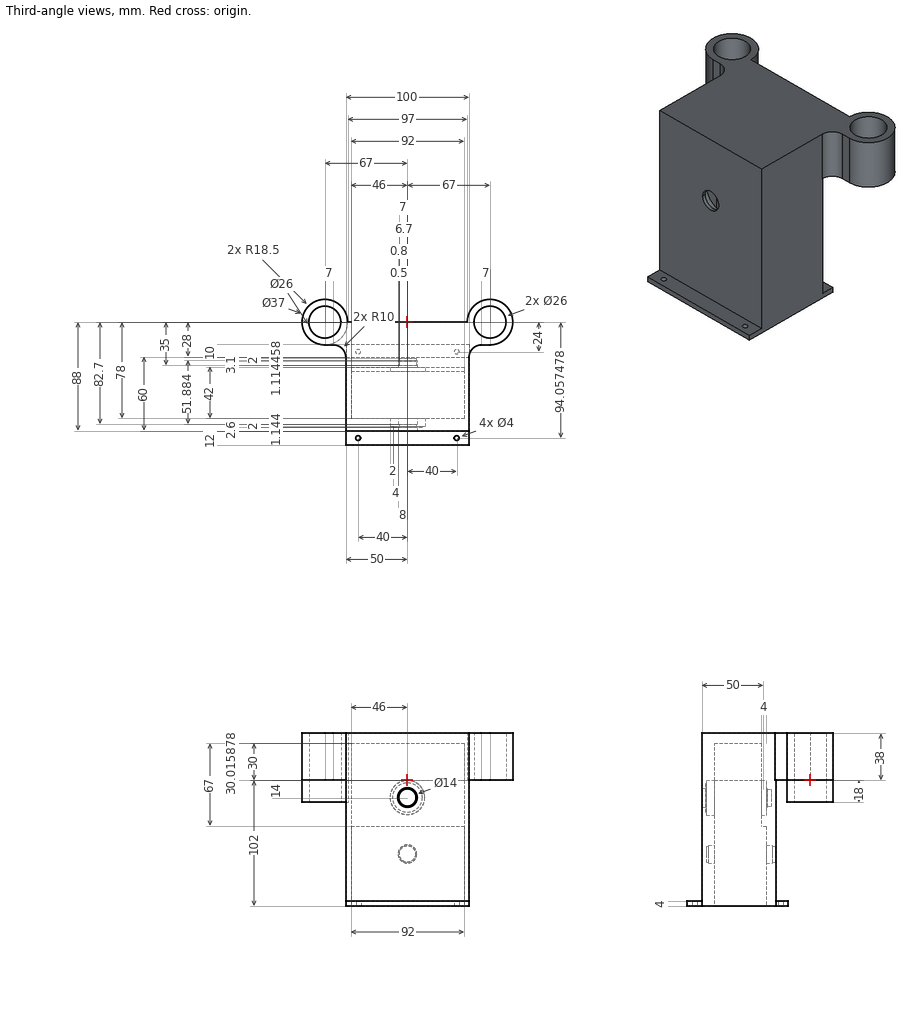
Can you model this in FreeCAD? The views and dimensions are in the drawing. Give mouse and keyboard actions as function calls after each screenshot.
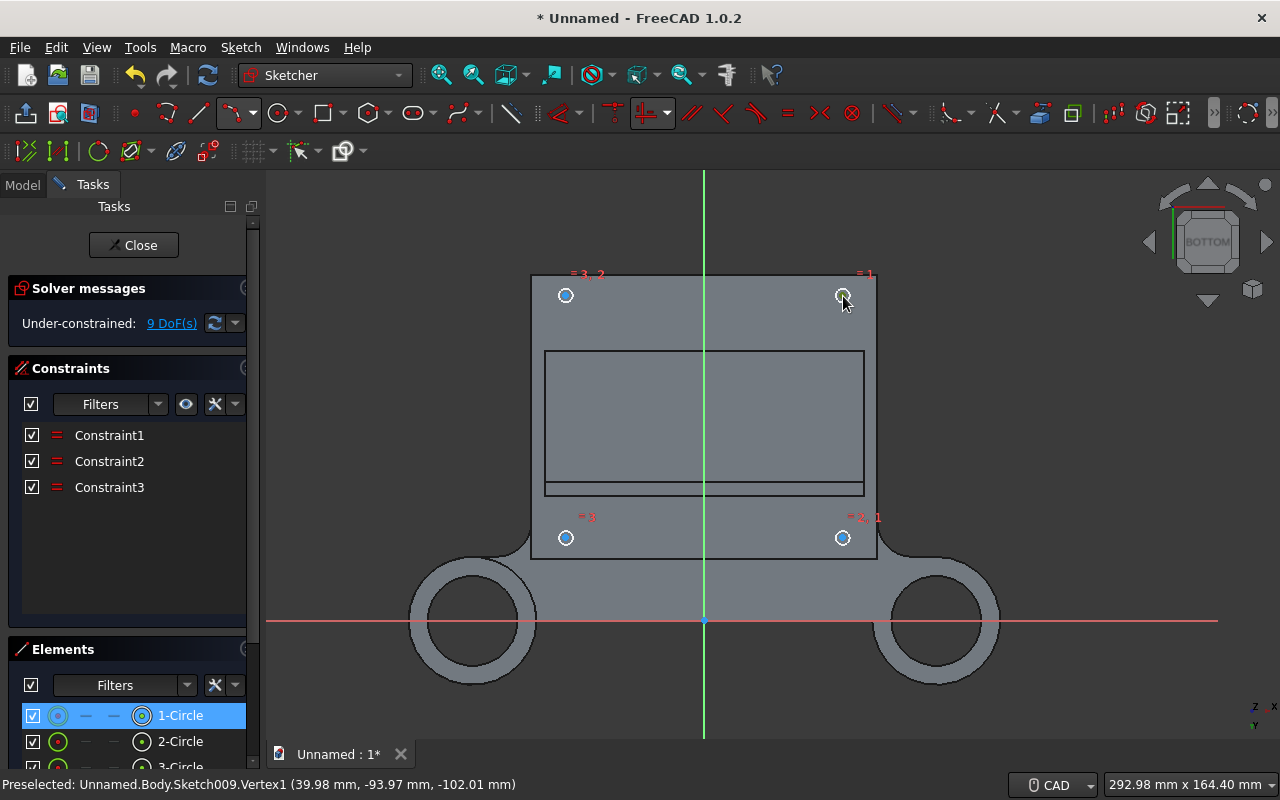
click(843, 538)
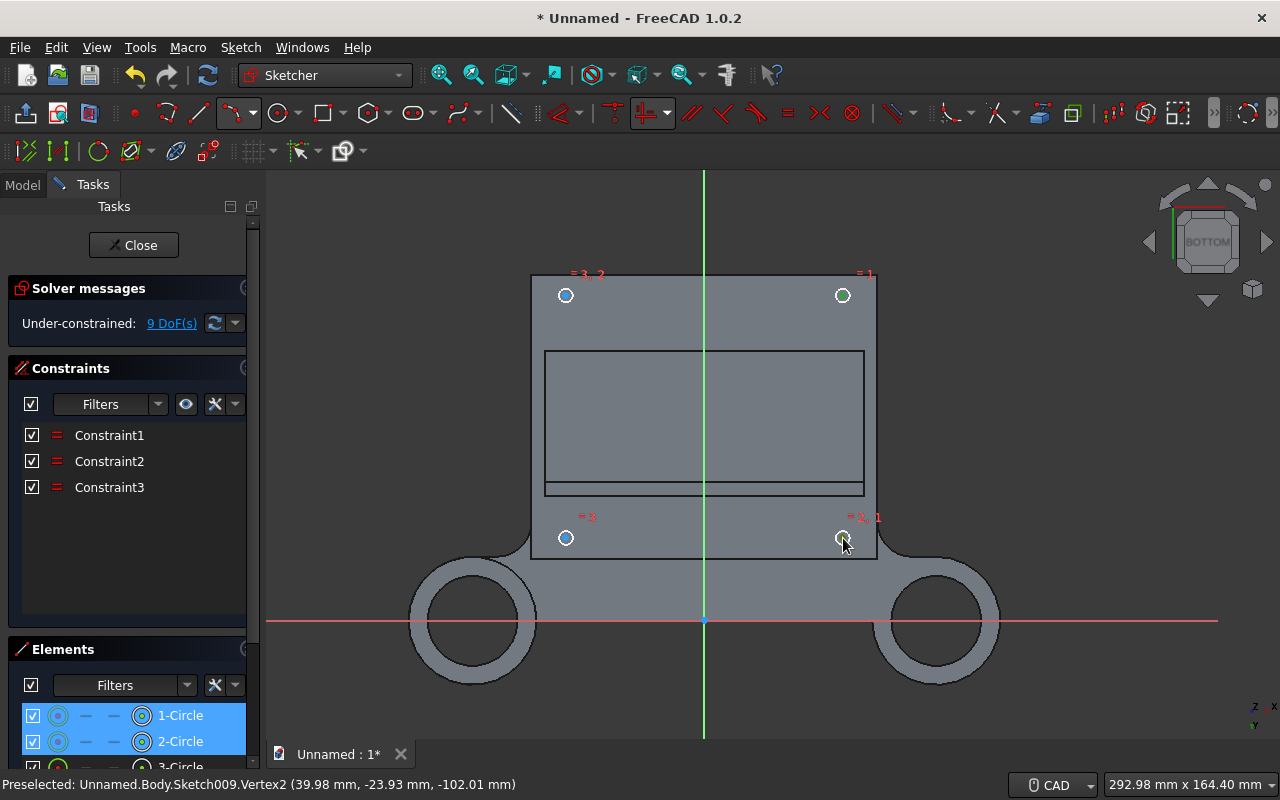
key(v)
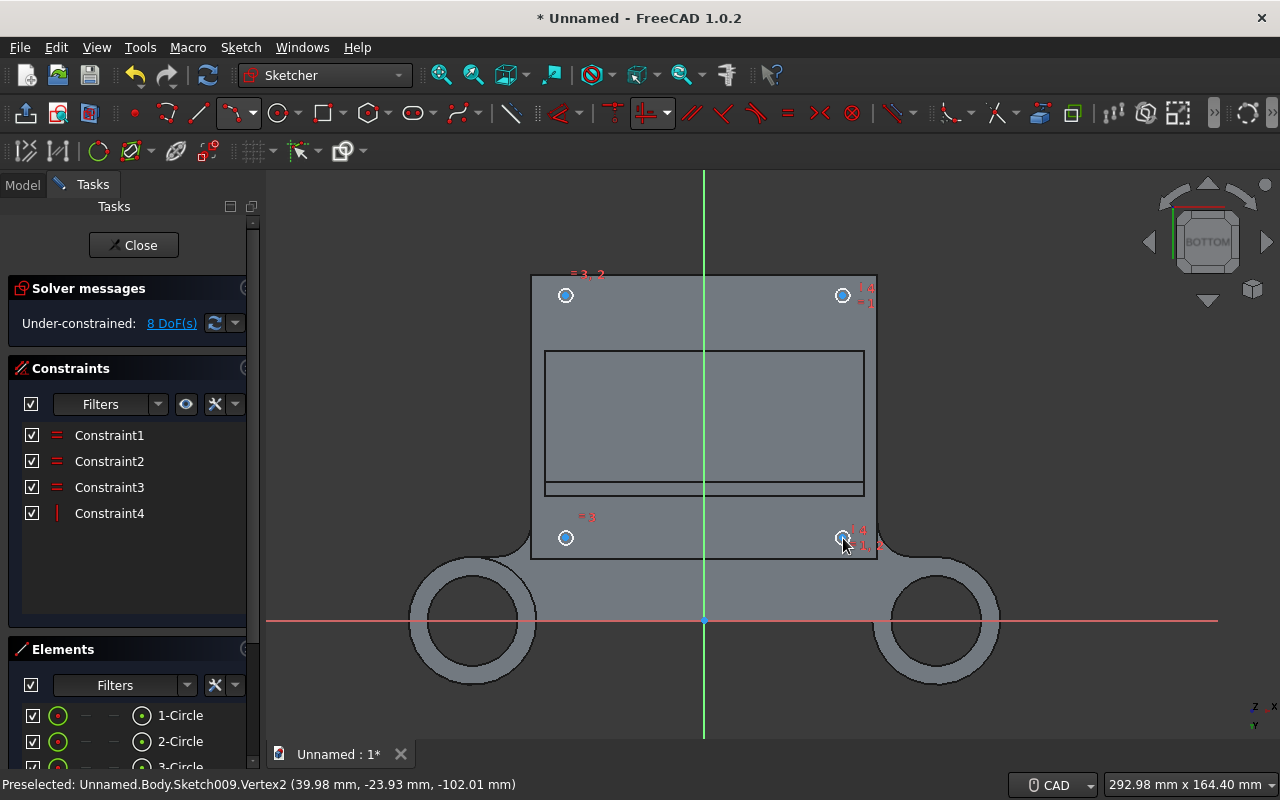
click(843, 296)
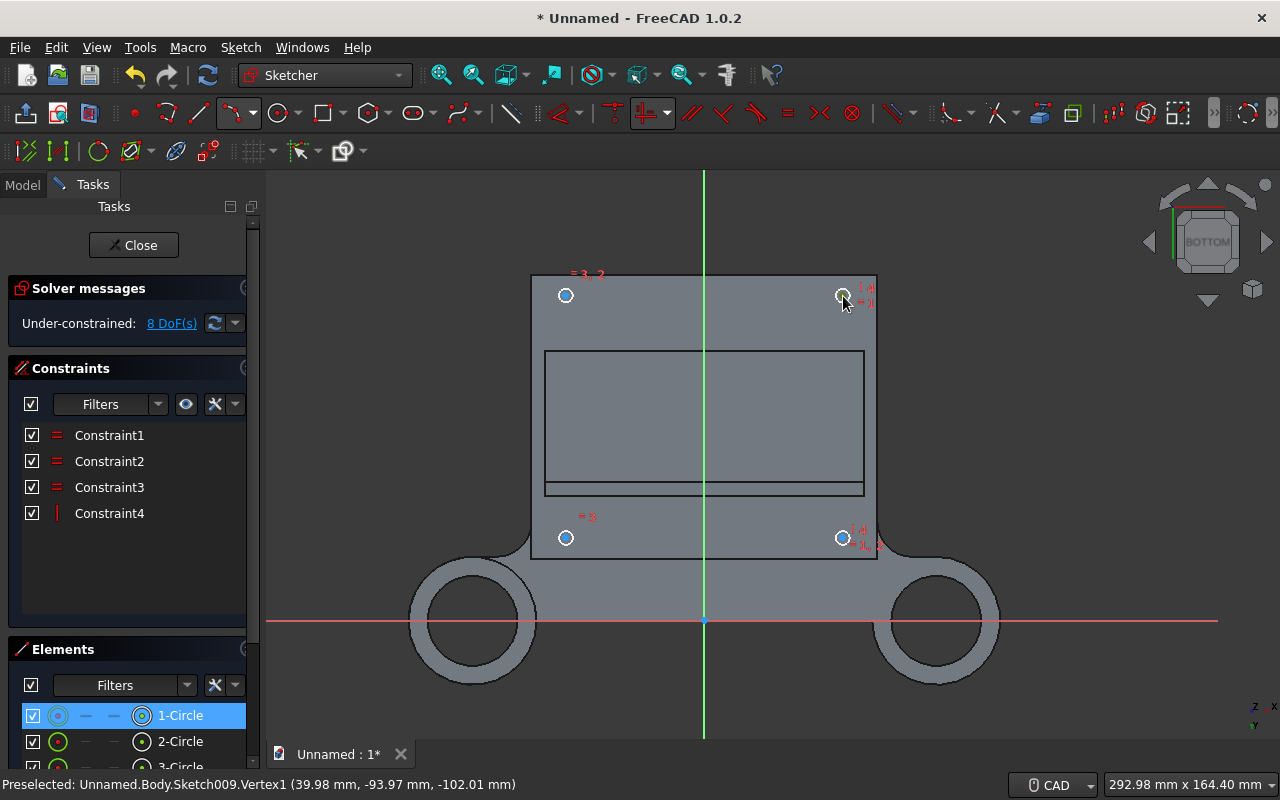
click(566, 296)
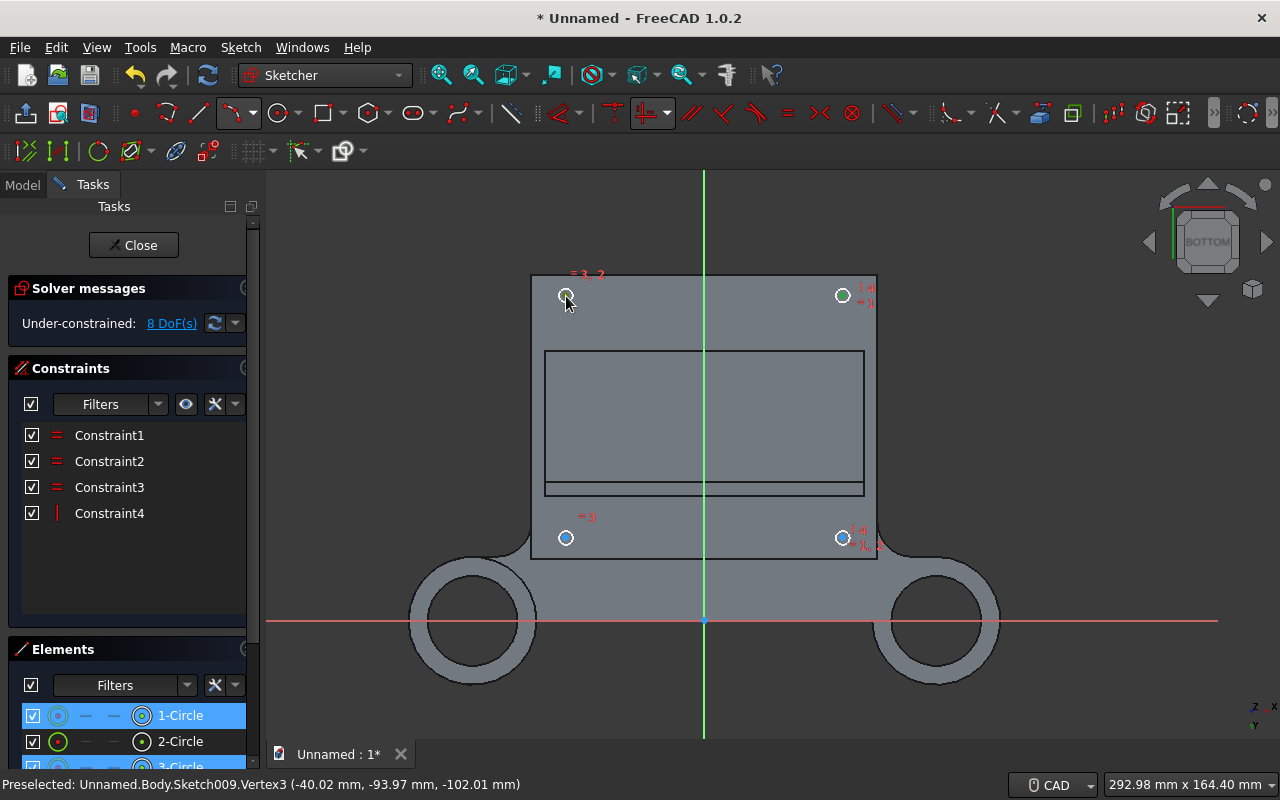
key(h)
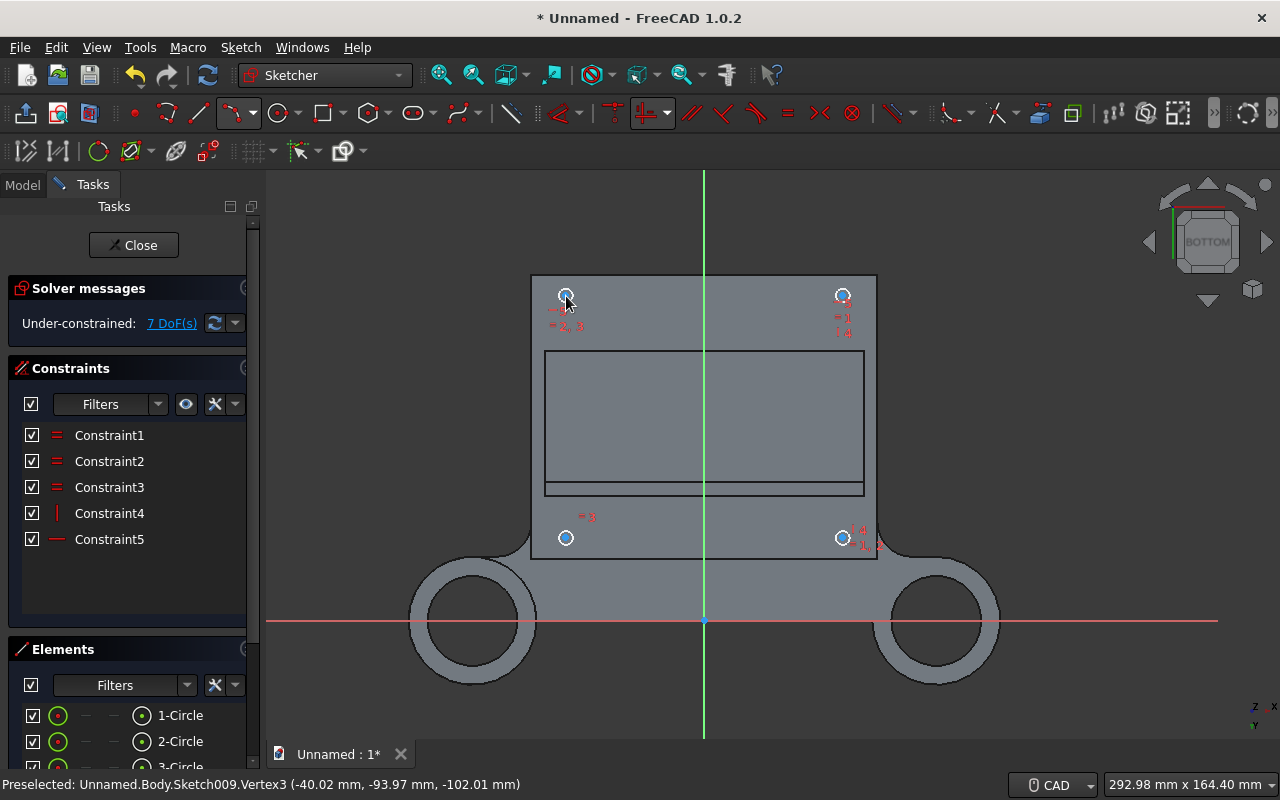
click(566, 296)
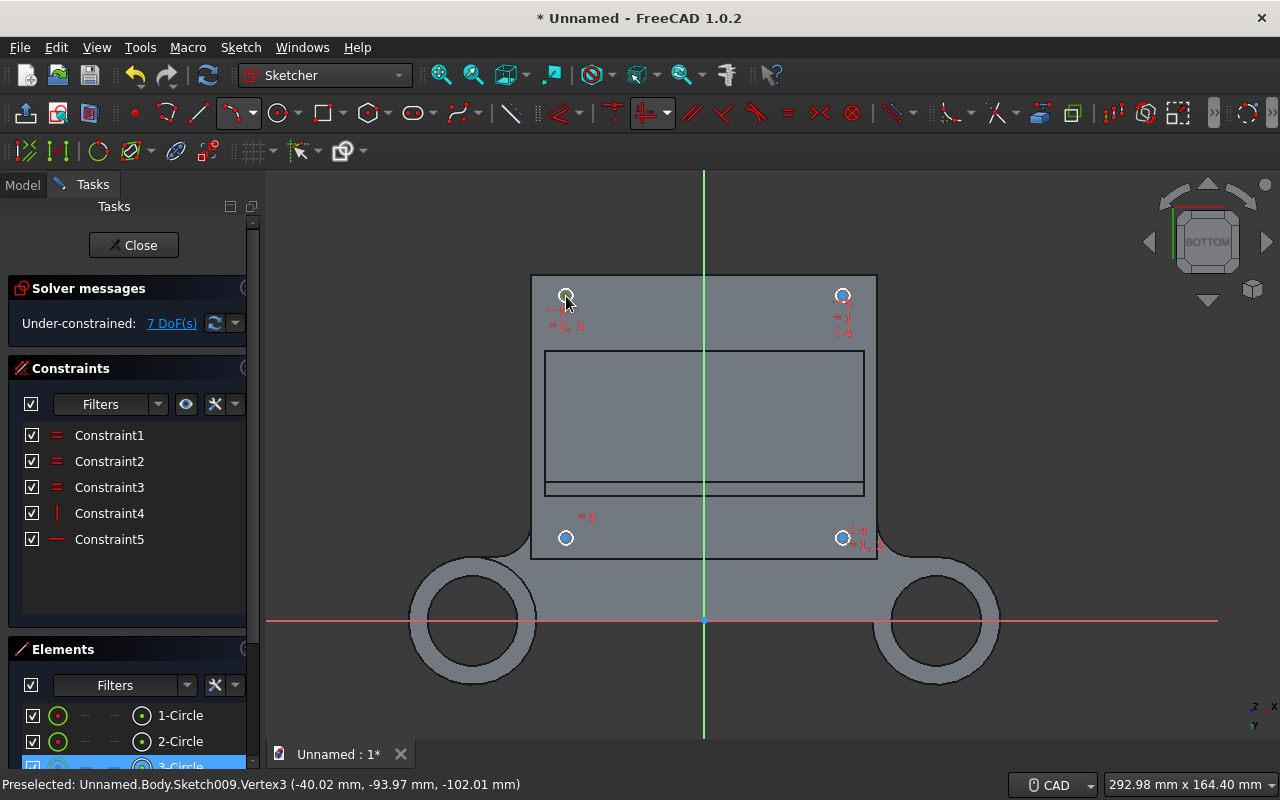
click(566, 538)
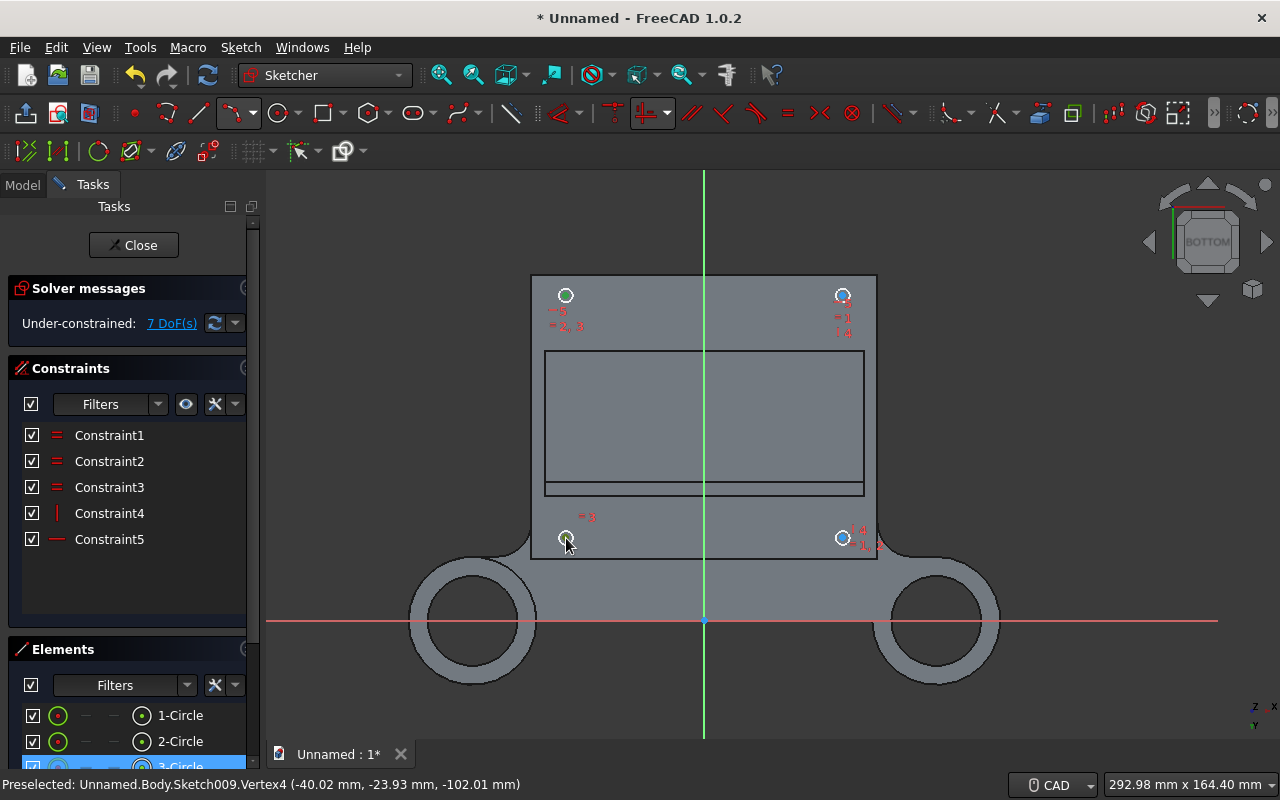
key(v)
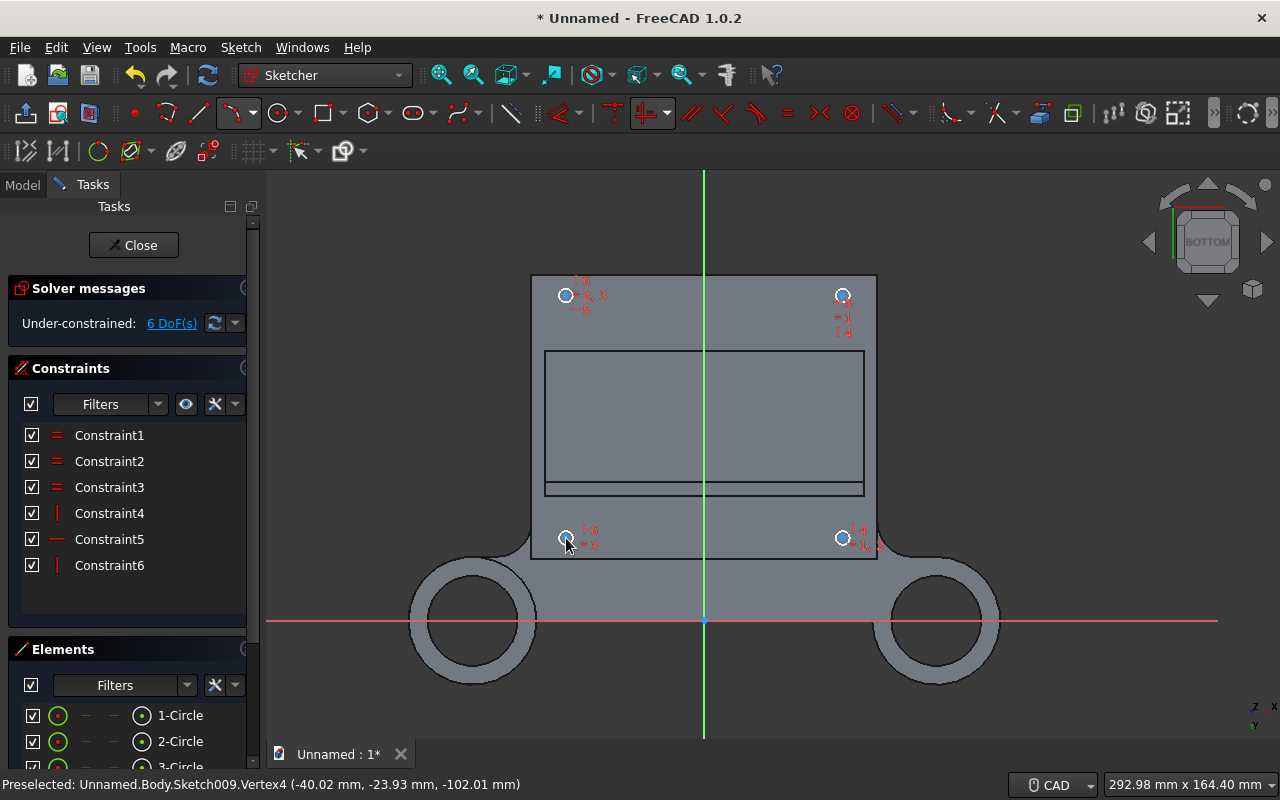
click(843, 538)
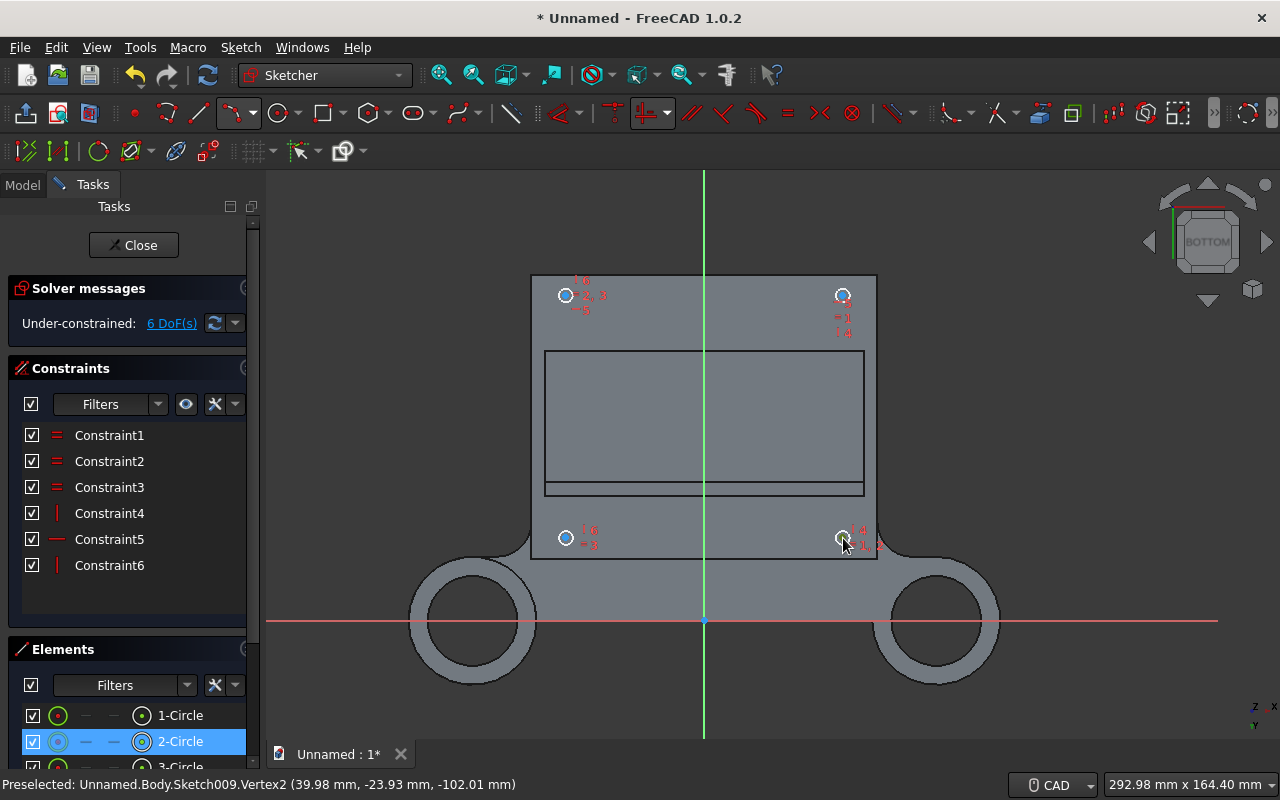
click(566, 538)